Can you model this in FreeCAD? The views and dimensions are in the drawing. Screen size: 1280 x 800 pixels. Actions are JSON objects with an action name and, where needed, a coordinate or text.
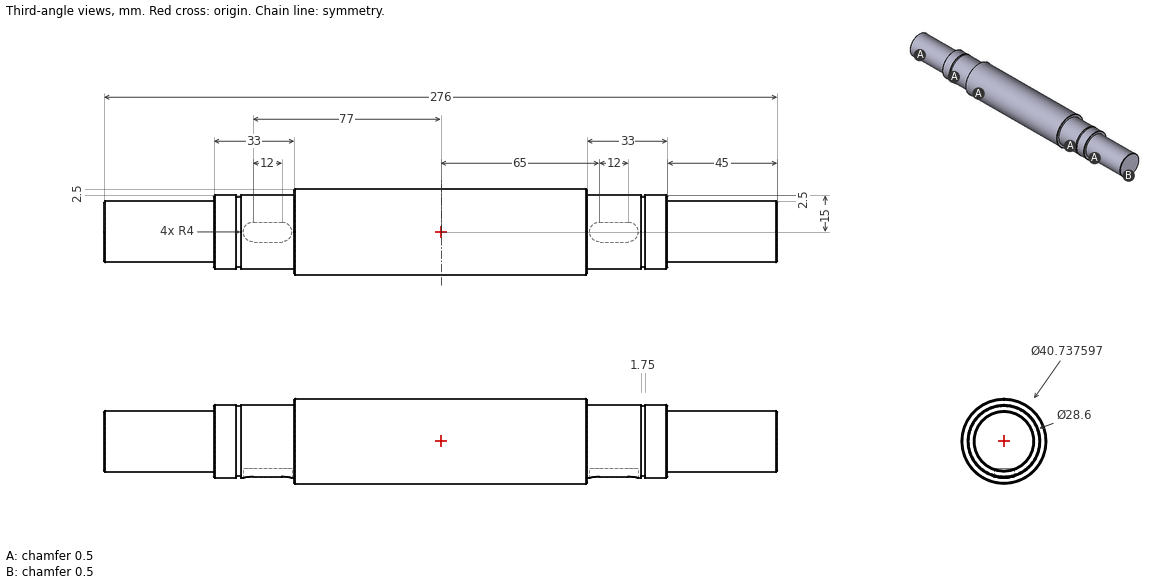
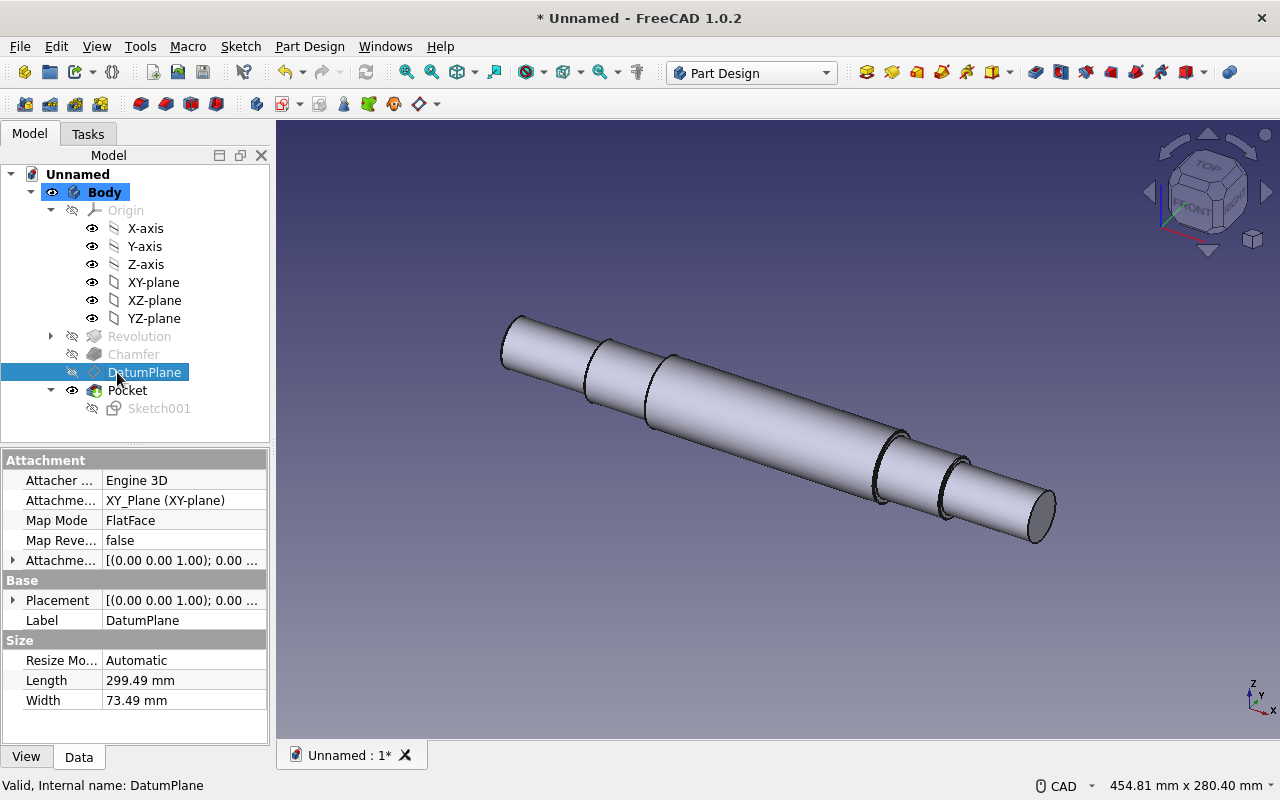
{"action": "left_click", "coordinate": [137, 318]}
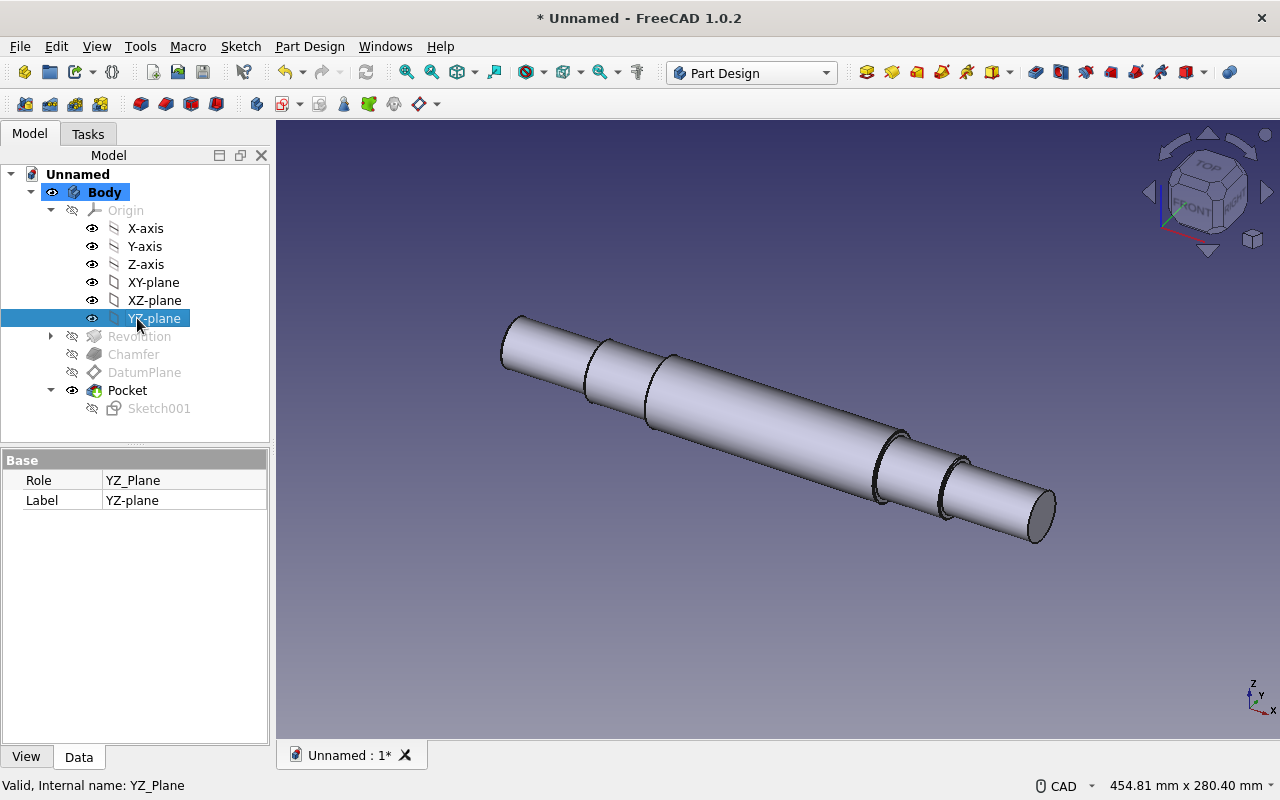
{"action": "left_click", "coordinate": [418, 104]}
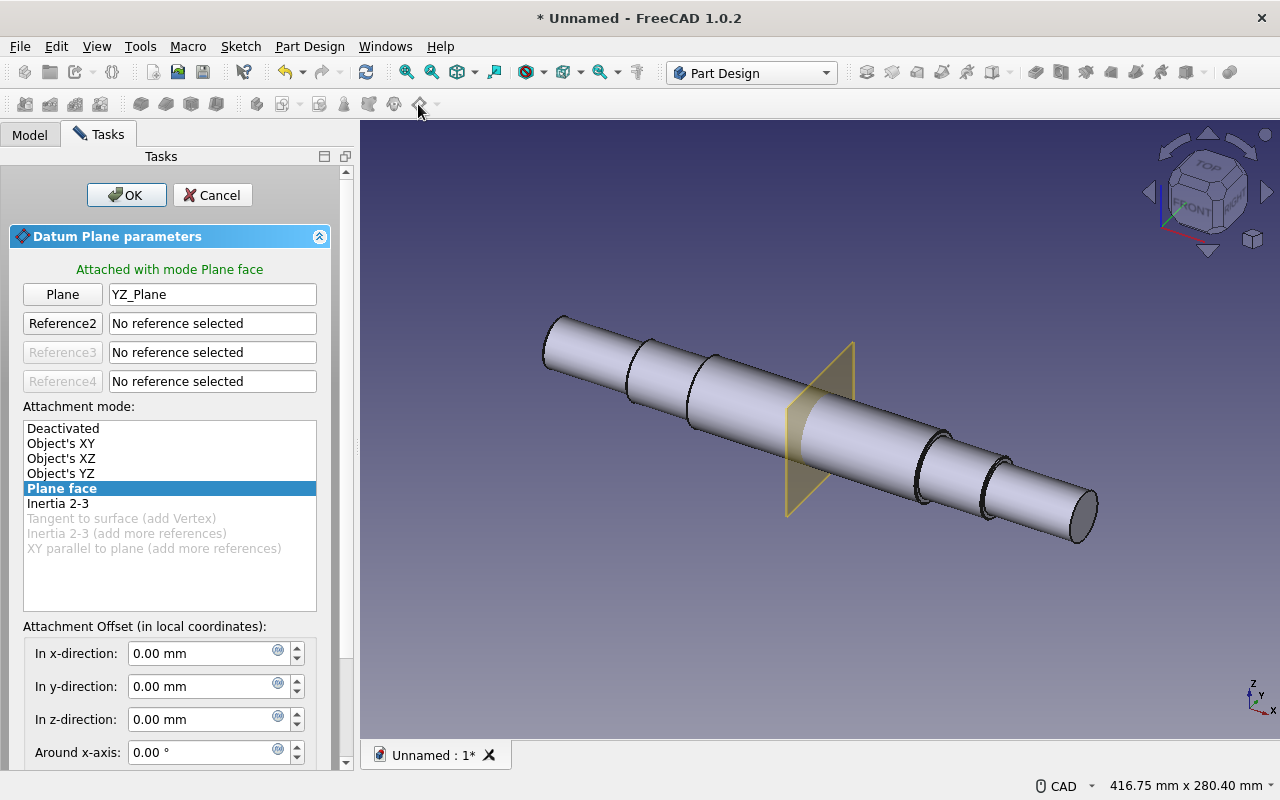
{"action": "triple_click", "coordinate": [210, 720]}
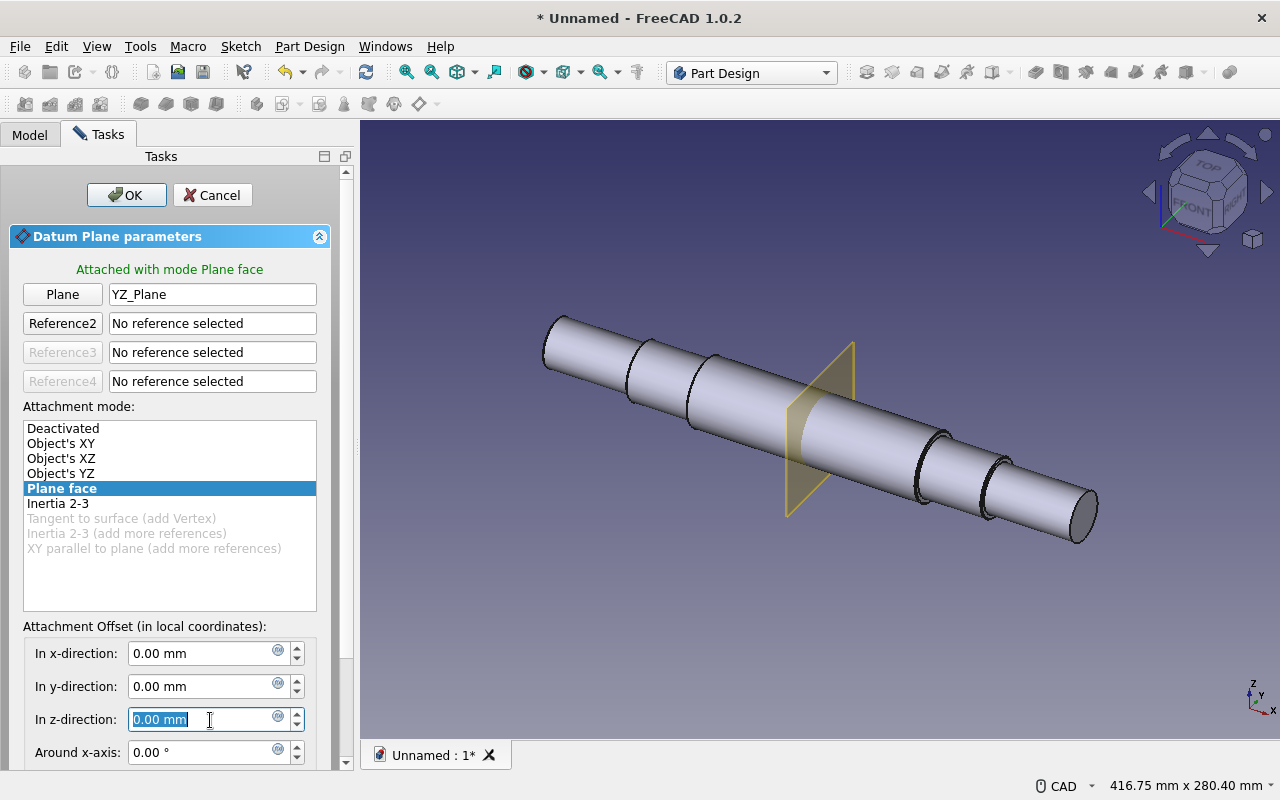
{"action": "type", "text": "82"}
{"action": "key", "text": "Tab"}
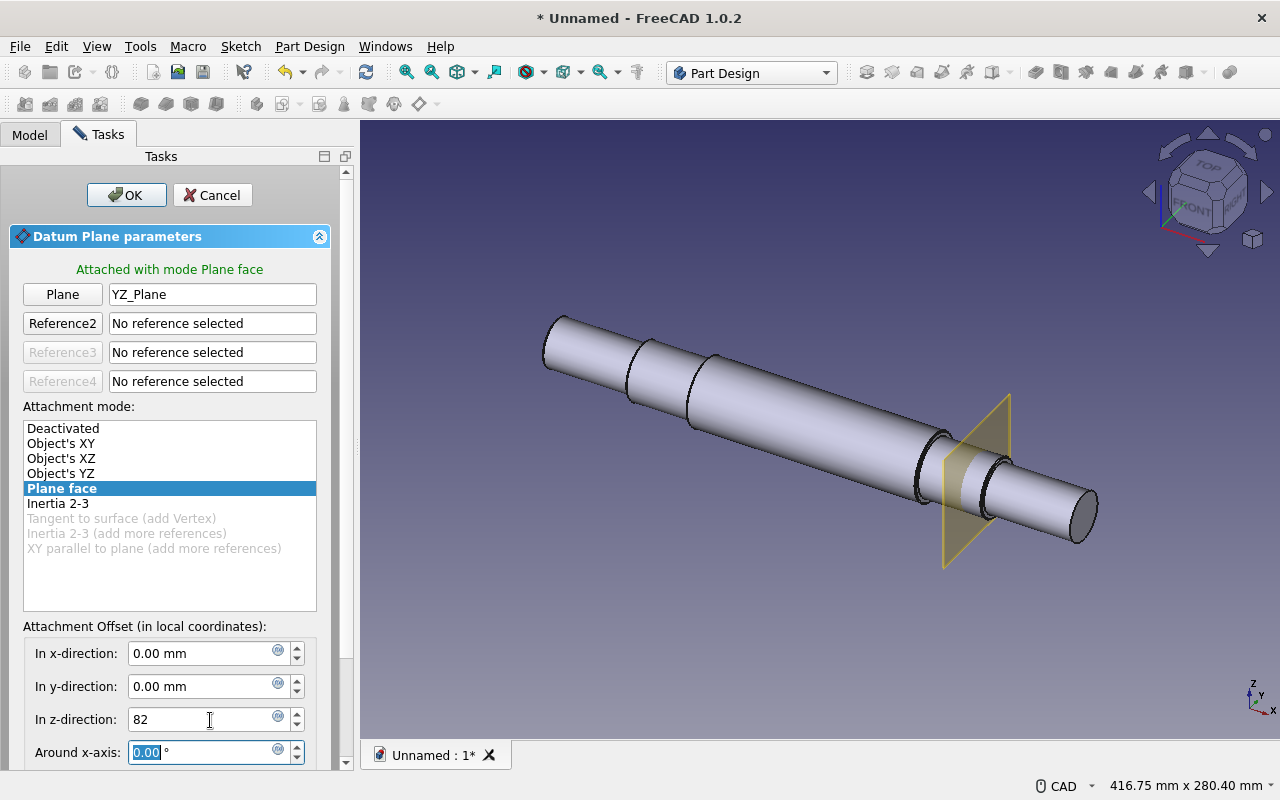
{"action": "left_click", "coordinate": [127, 195]}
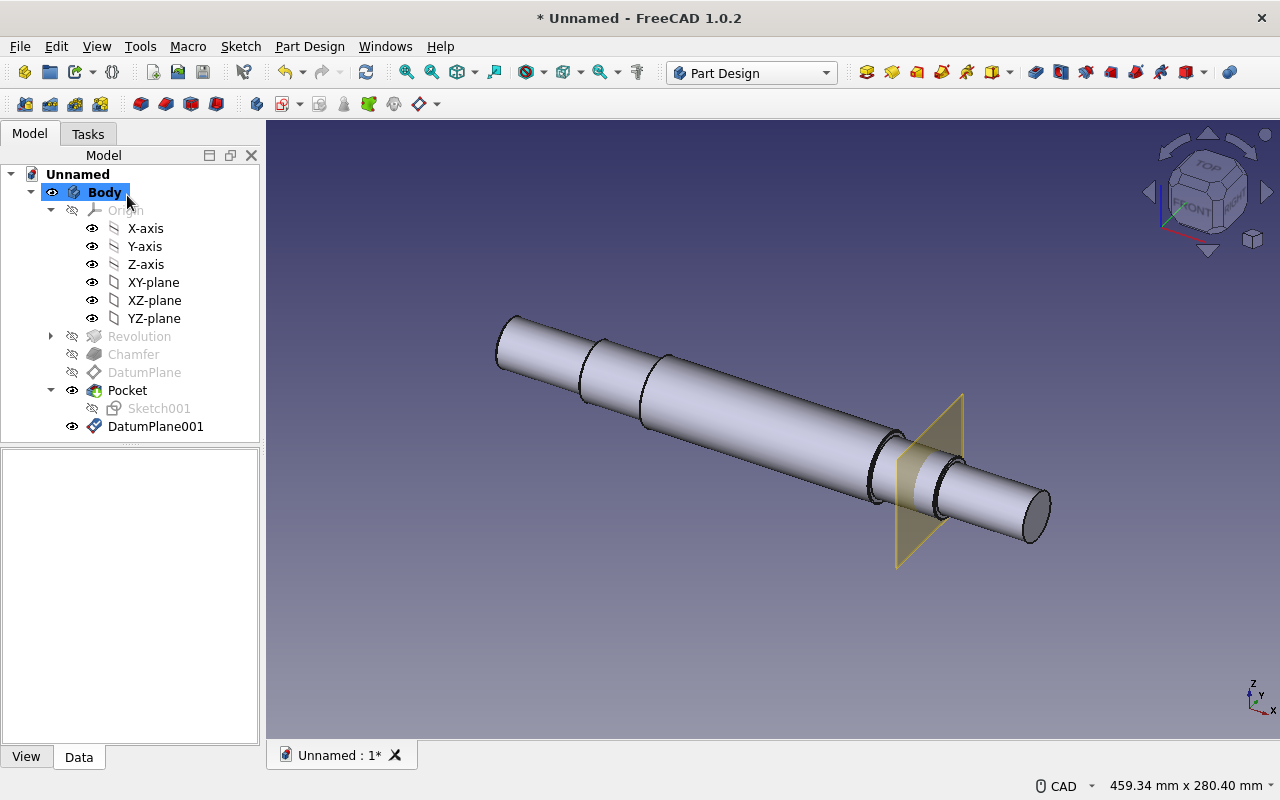
{"action": "left_click", "coordinate": [117, 426]}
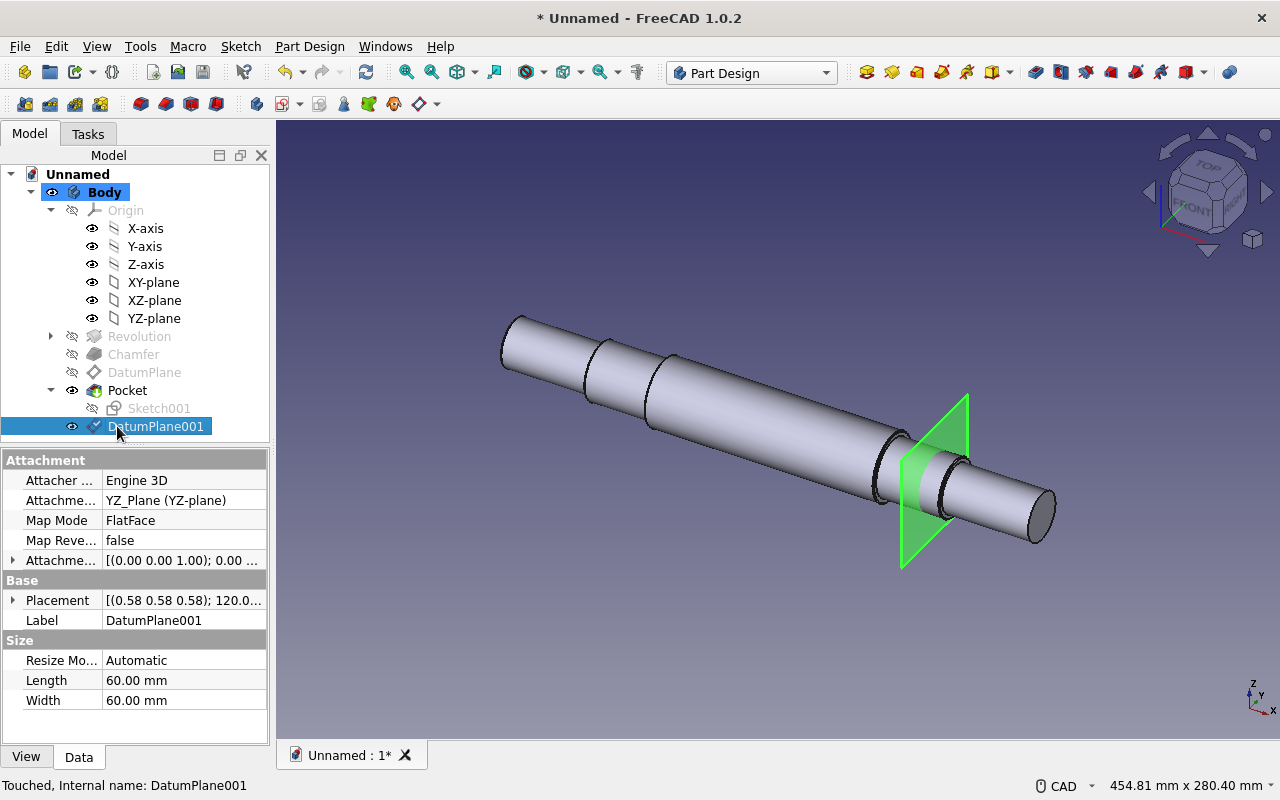
{"action": "left_click", "coordinate": [282, 104]}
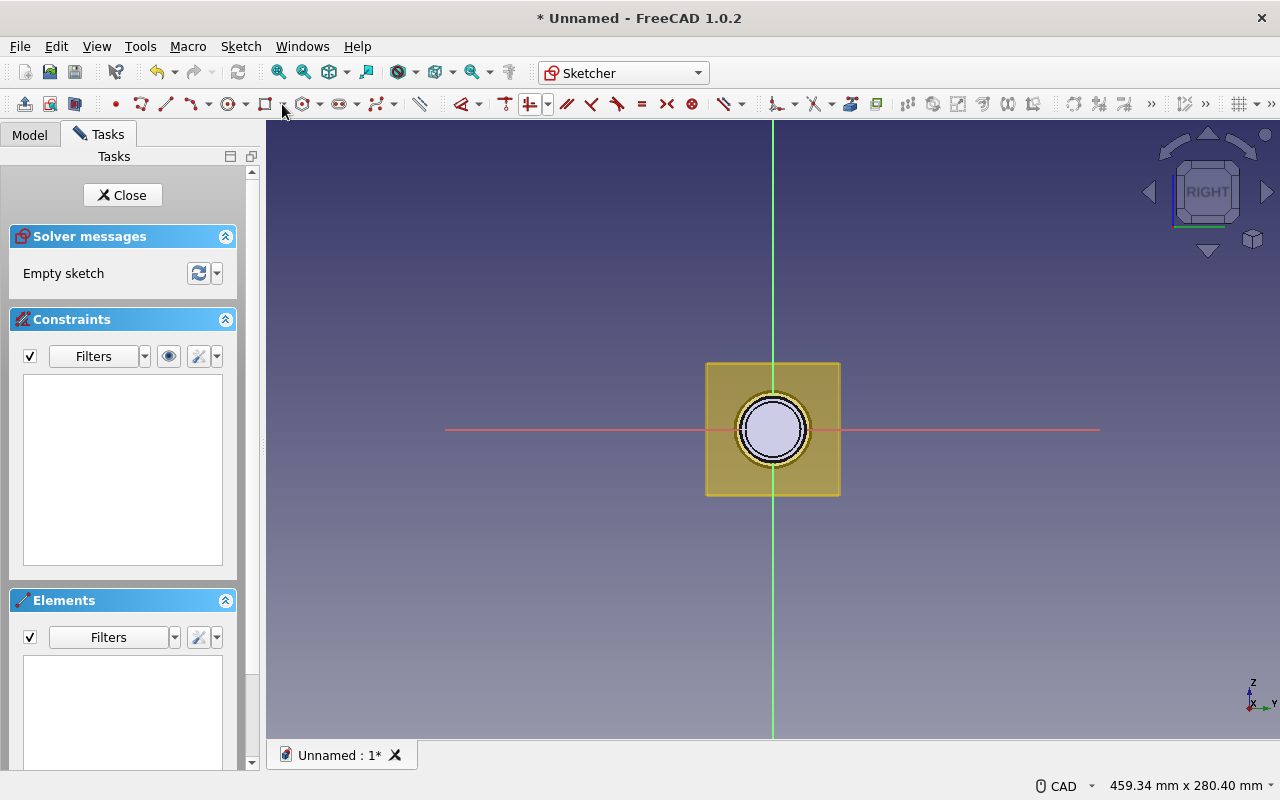
{"action": "left_click", "coordinate": [75, 104]}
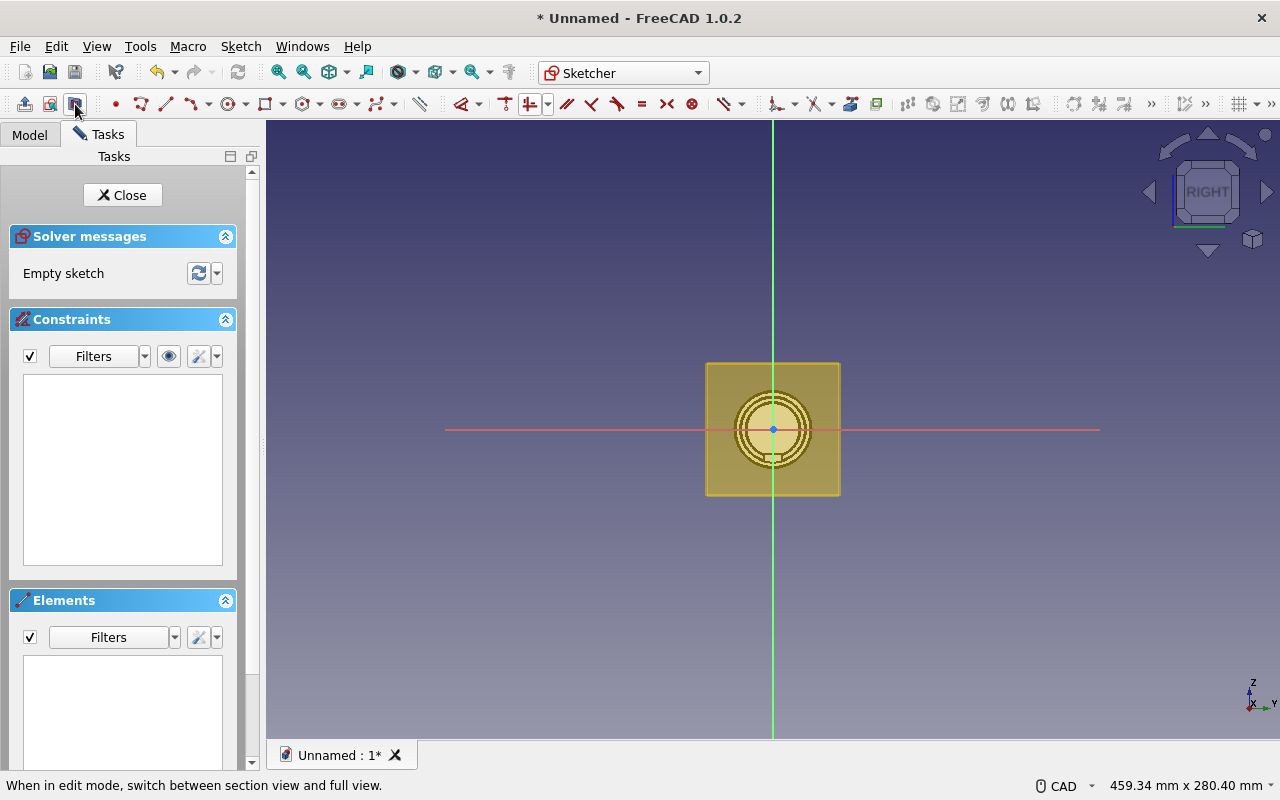
{"action": "scroll", "coordinate": [795, 430], "scroll_direction": "up", "scroll_amount": 7}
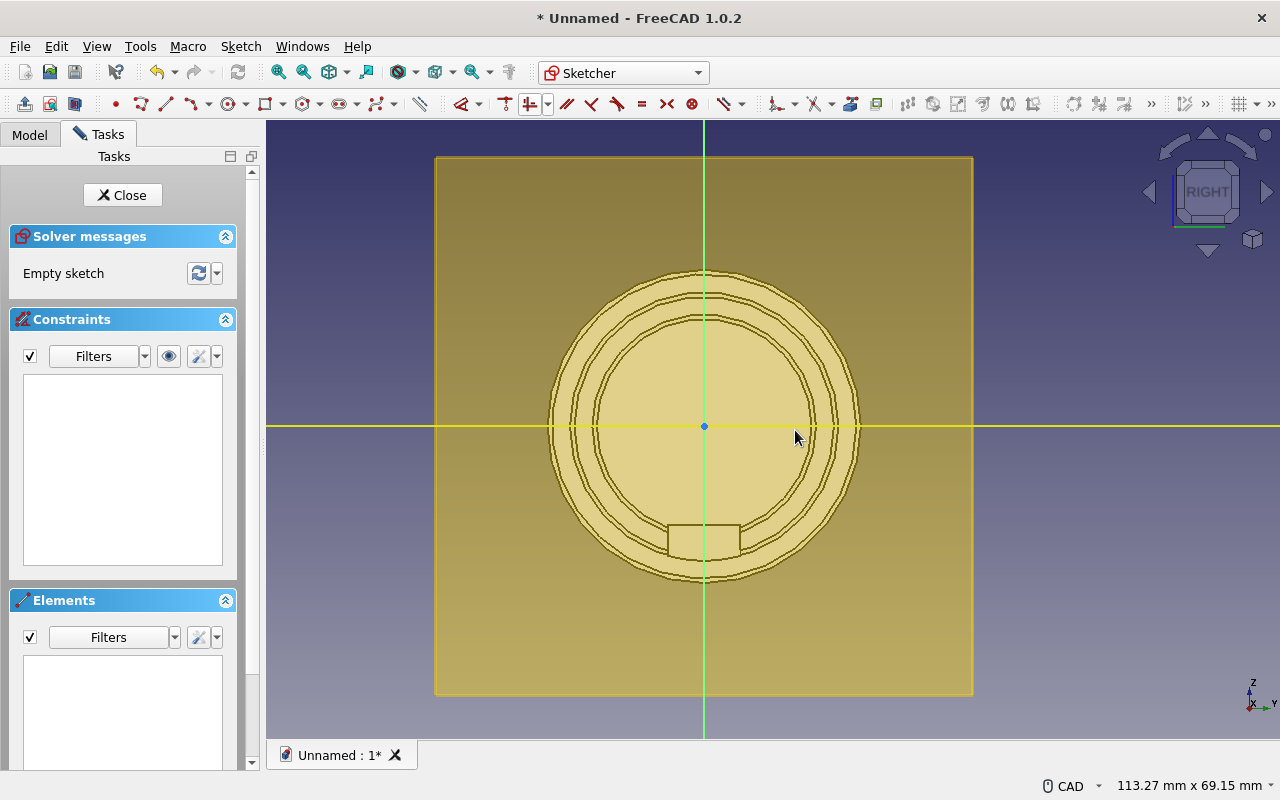
{"action": "left_click", "coordinate": [228, 104]}